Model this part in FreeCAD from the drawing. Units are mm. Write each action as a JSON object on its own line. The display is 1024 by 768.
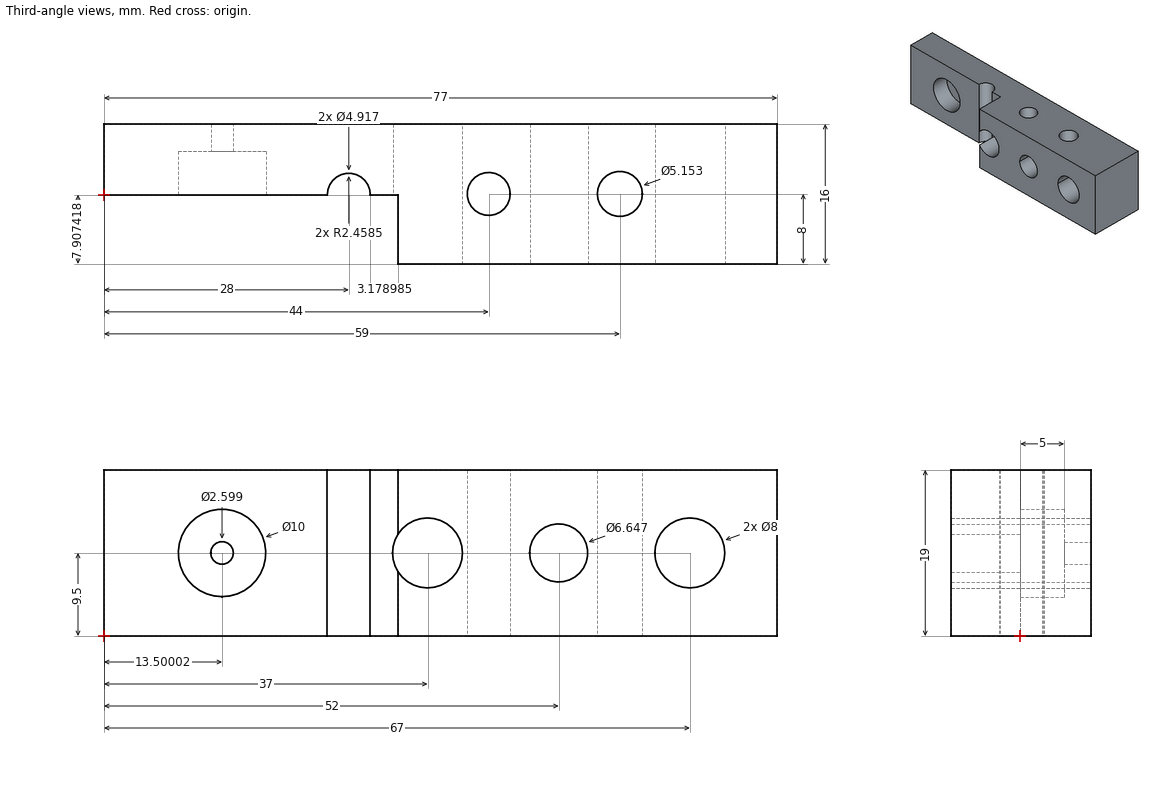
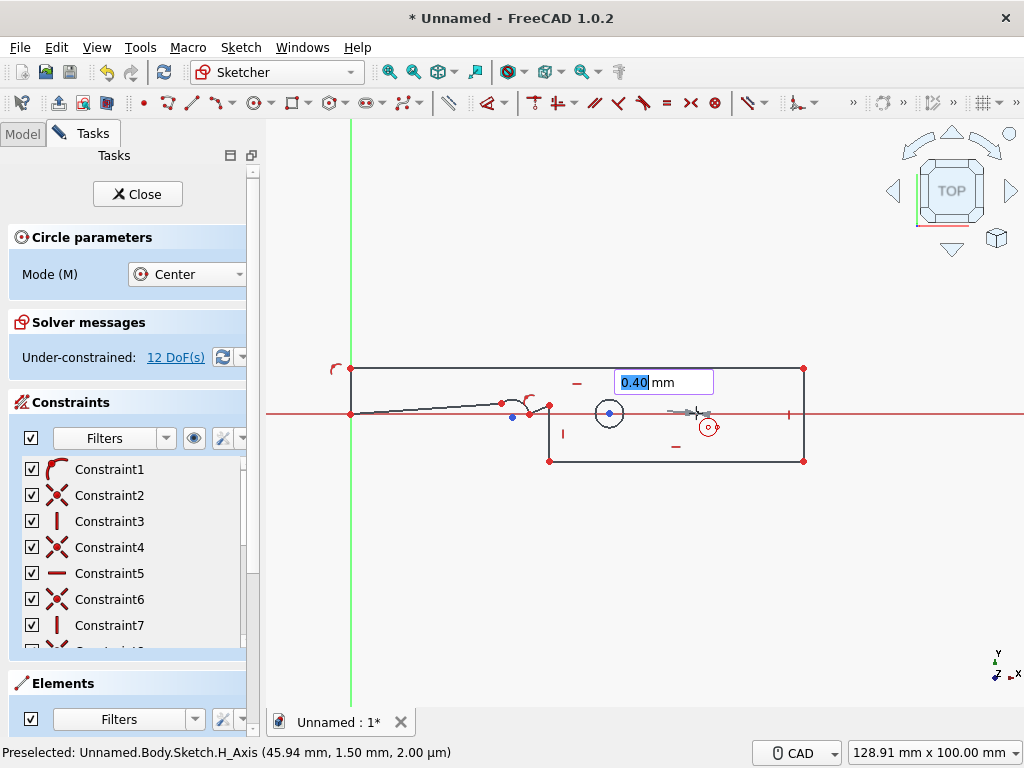
{"action": "scroll", "coordinate": [708, 403], "scroll_direction": "up", "scroll_amount": 2}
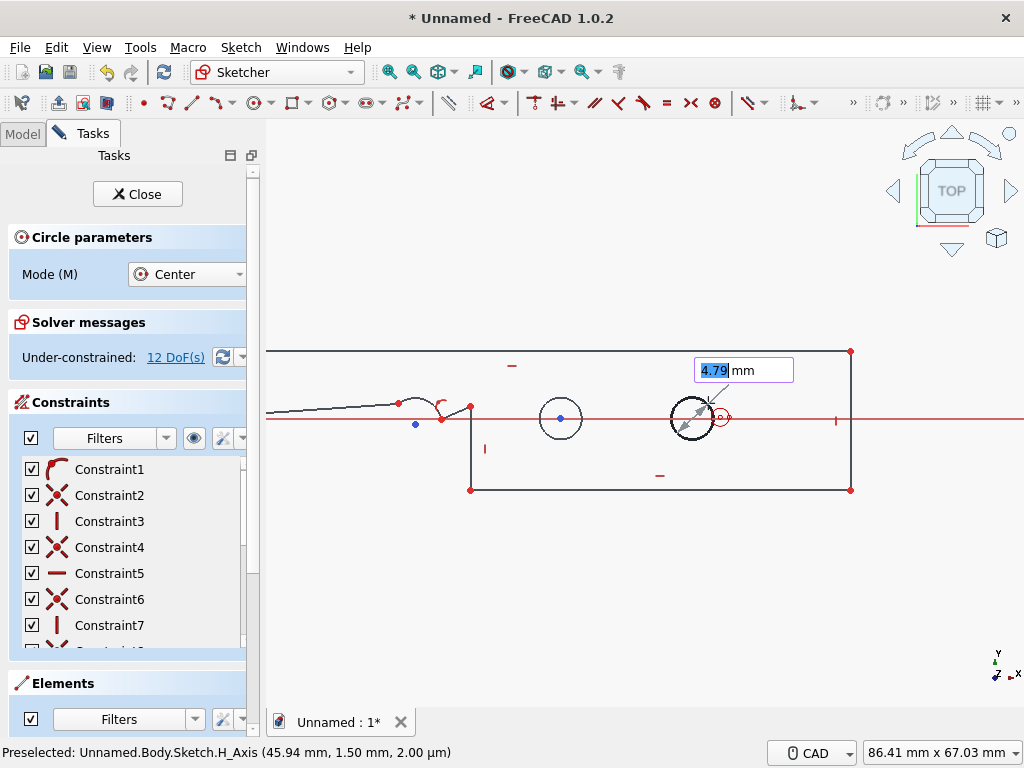
{"action": "left_click", "coordinate": [708, 403]}
{"action": "key", "text": "Escape"}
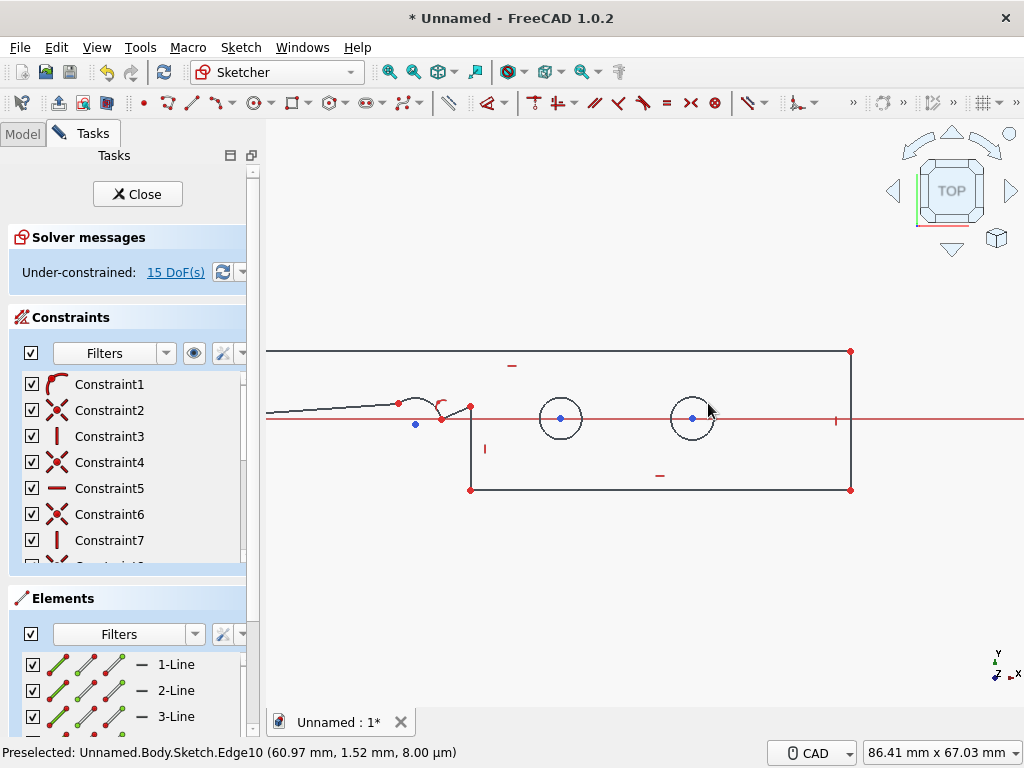
{"action": "scroll", "coordinate": [450, 416], "scroll_direction": "up", "scroll_amount": 2}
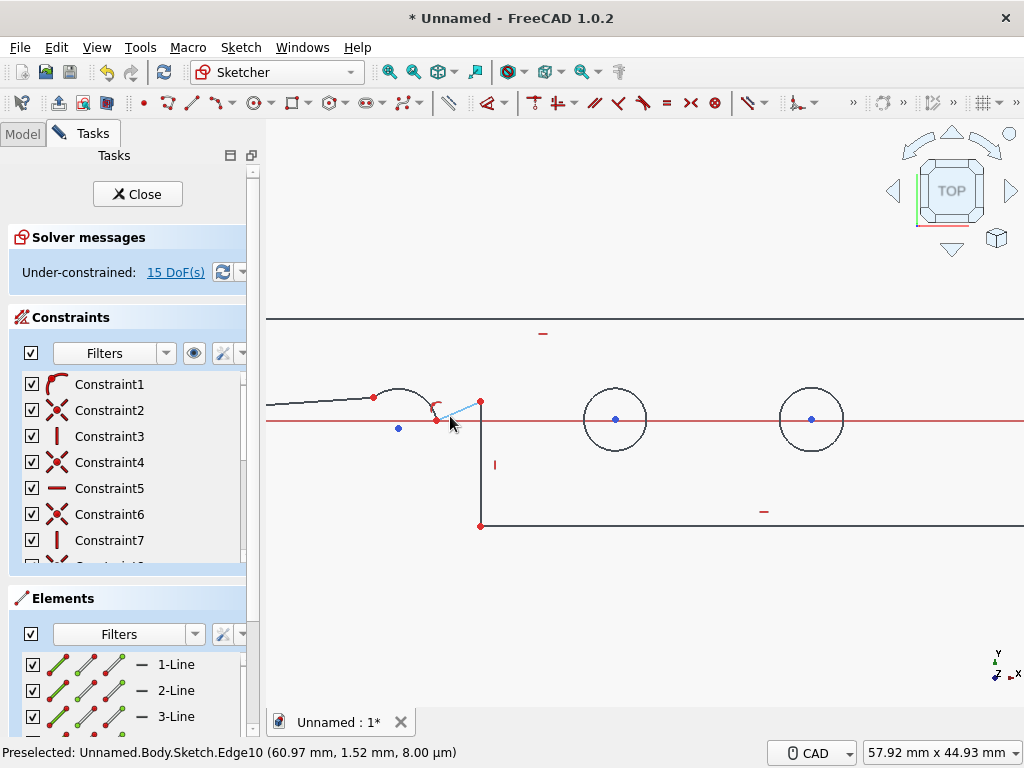
{"action": "left_click", "coordinate": [450, 415]}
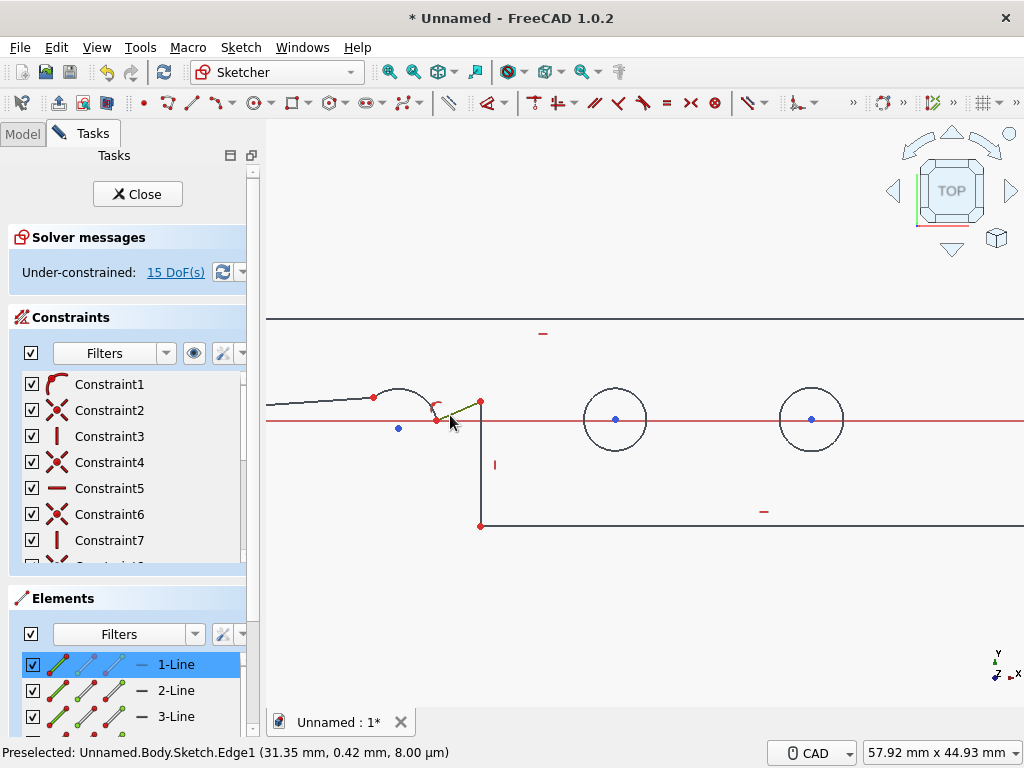
{"action": "key", "text": "h"}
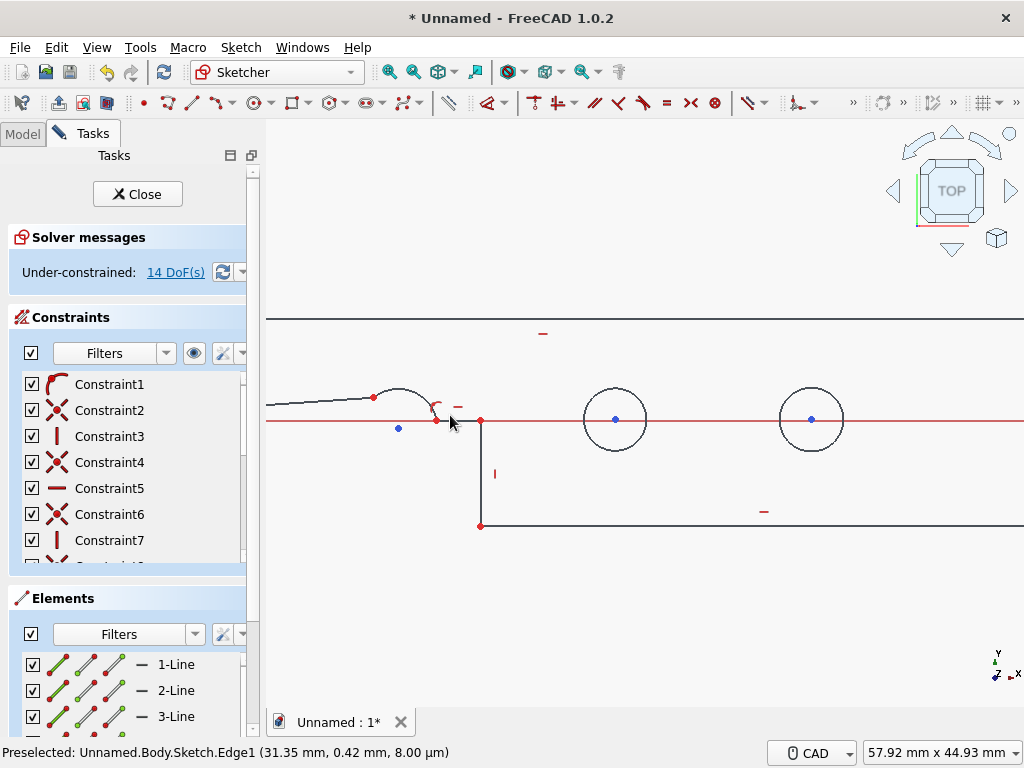
{"action": "left_click", "coordinate": [307, 402]}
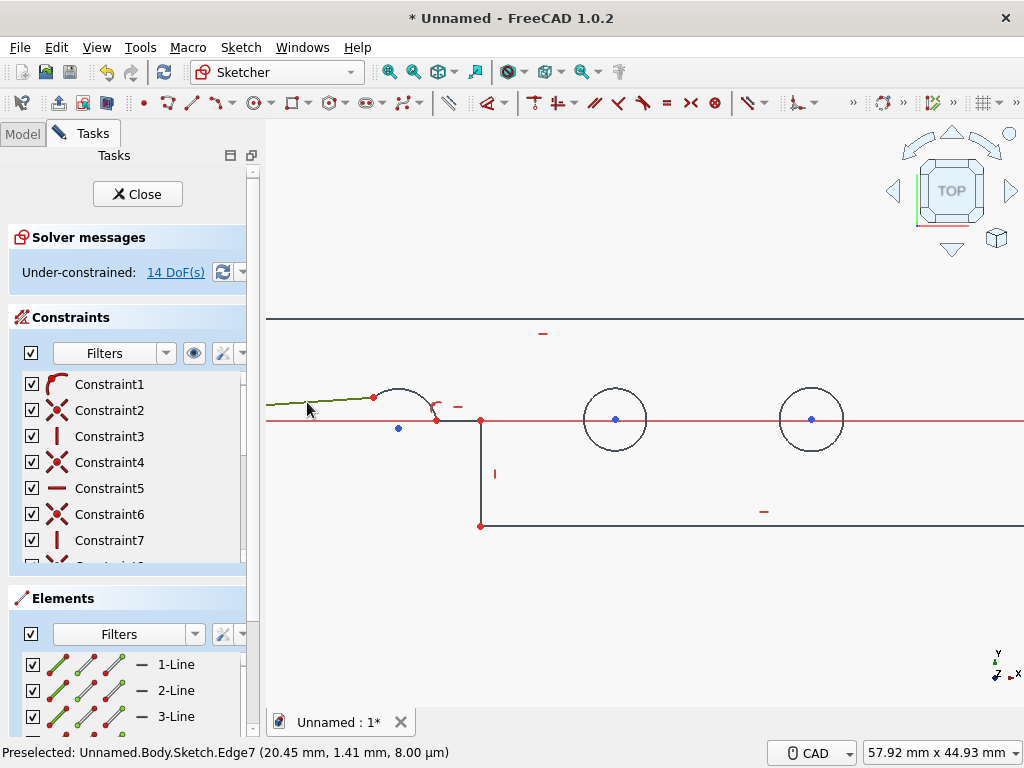
{"action": "key", "text": "h"}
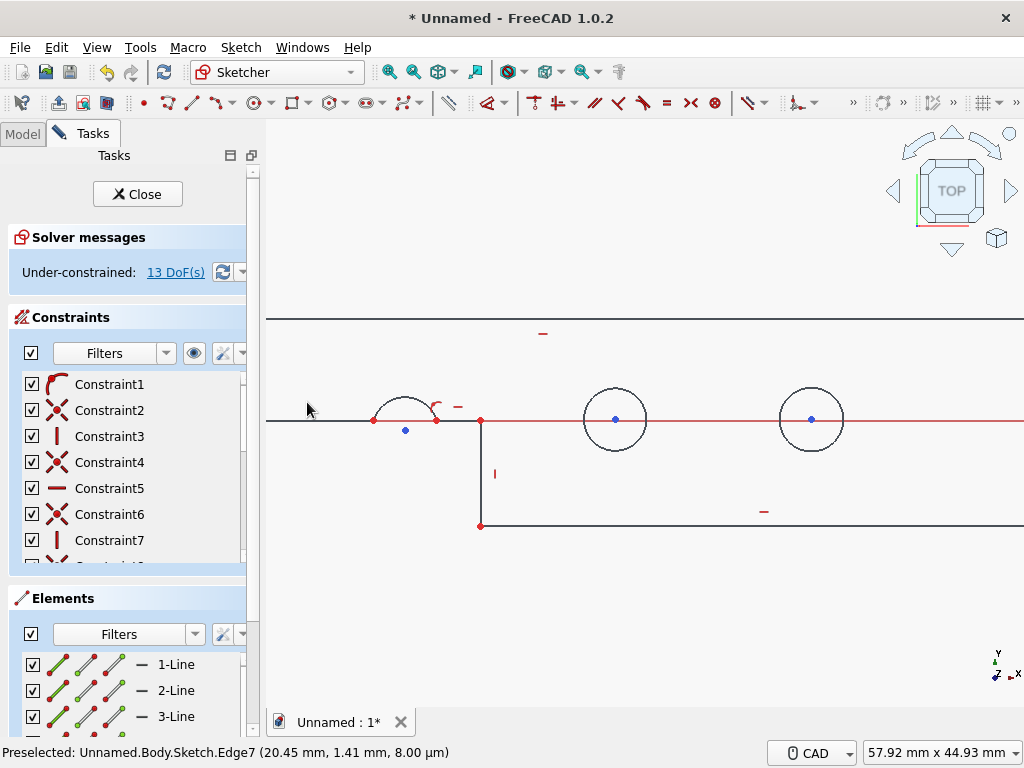
{"action": "left_click", "coordinate": [405, 430]}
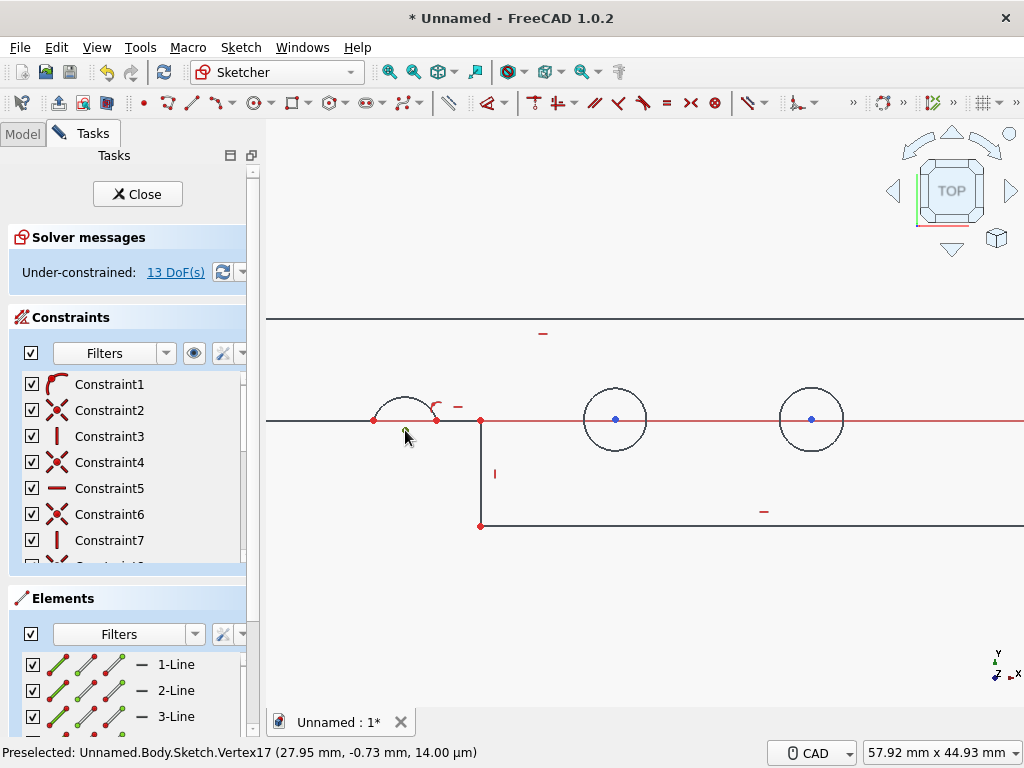
{"action": "left_click", "coordinate": [536, 421]}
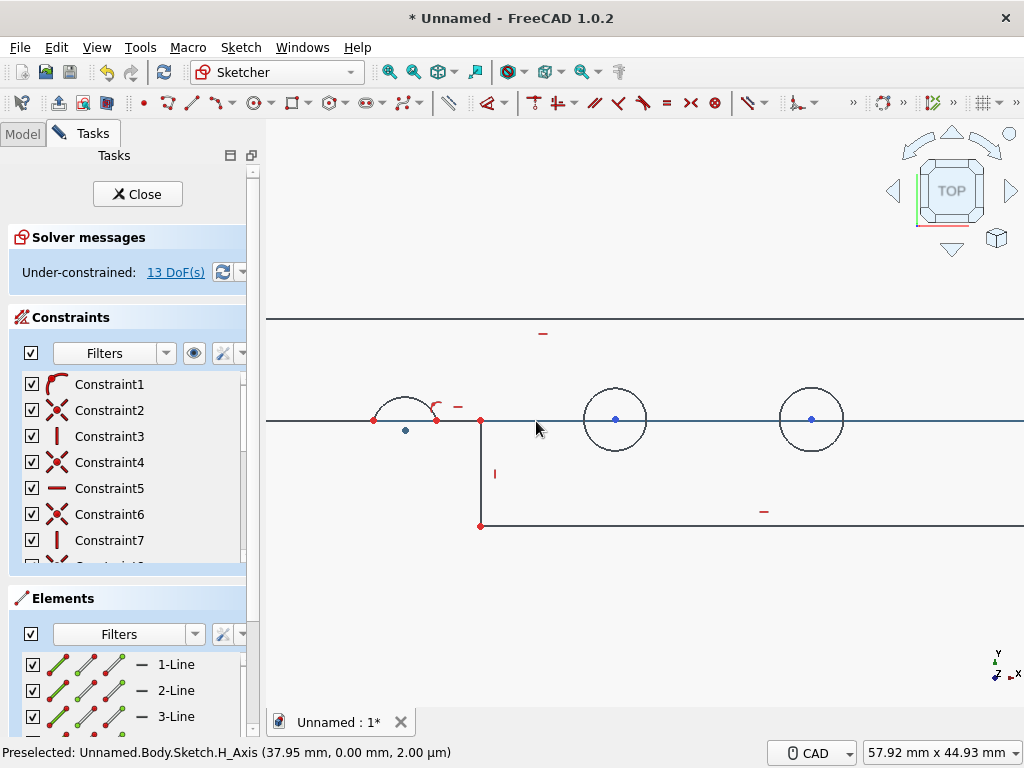
{"action": "key", "text": "c"}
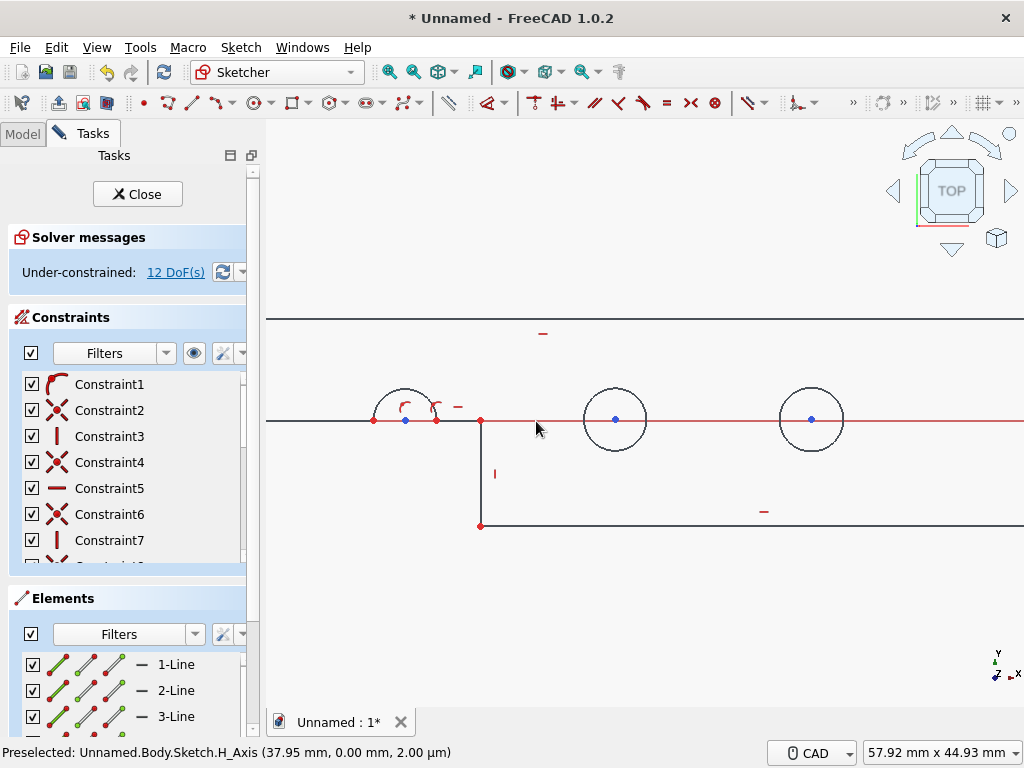
{"action": "left_click", "coordinate": [615, 420]}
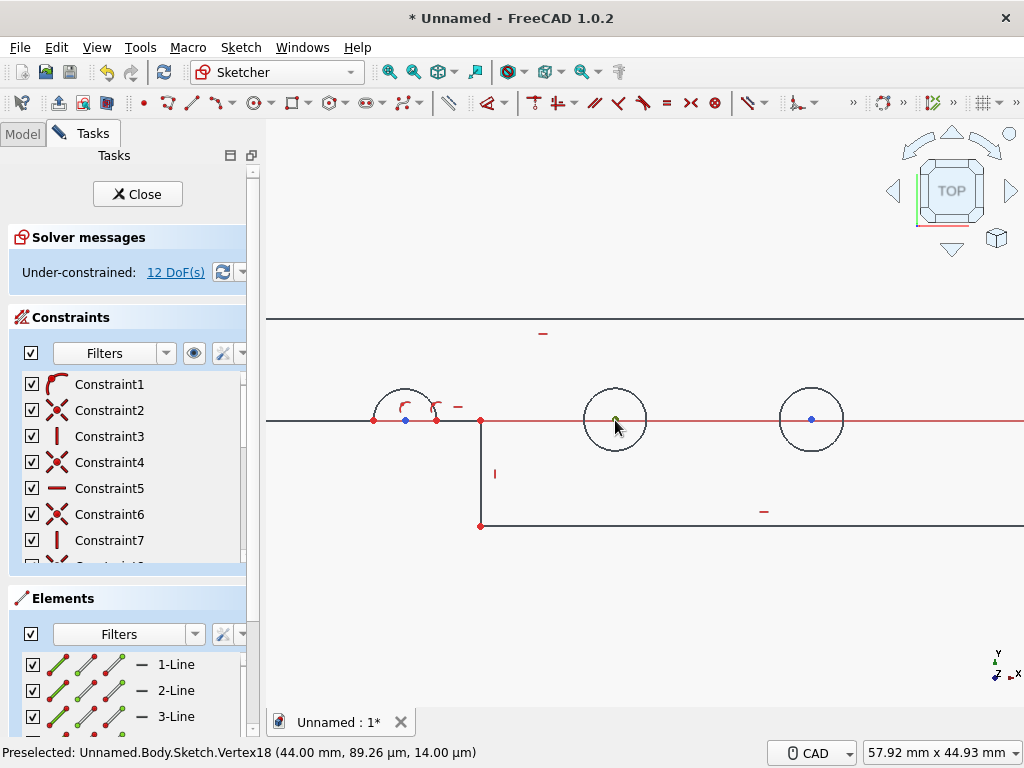
{"action": "left_click", "coordinate": [811, 420]}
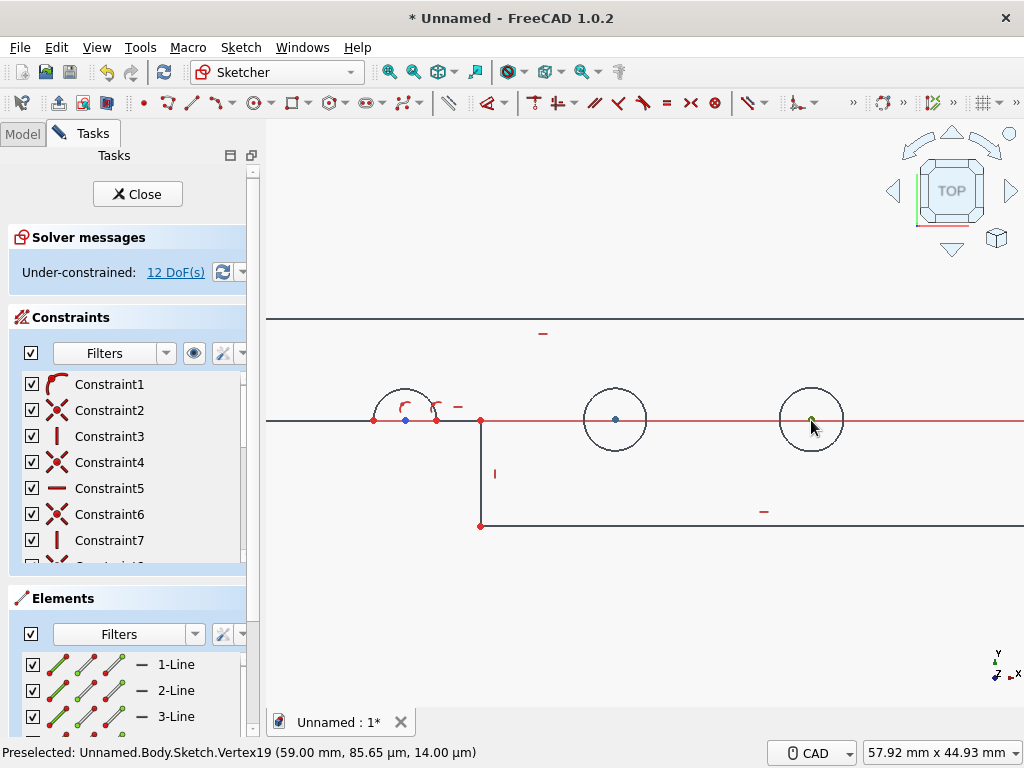
{"action": "left_click", "coordinate": [576, 104]}